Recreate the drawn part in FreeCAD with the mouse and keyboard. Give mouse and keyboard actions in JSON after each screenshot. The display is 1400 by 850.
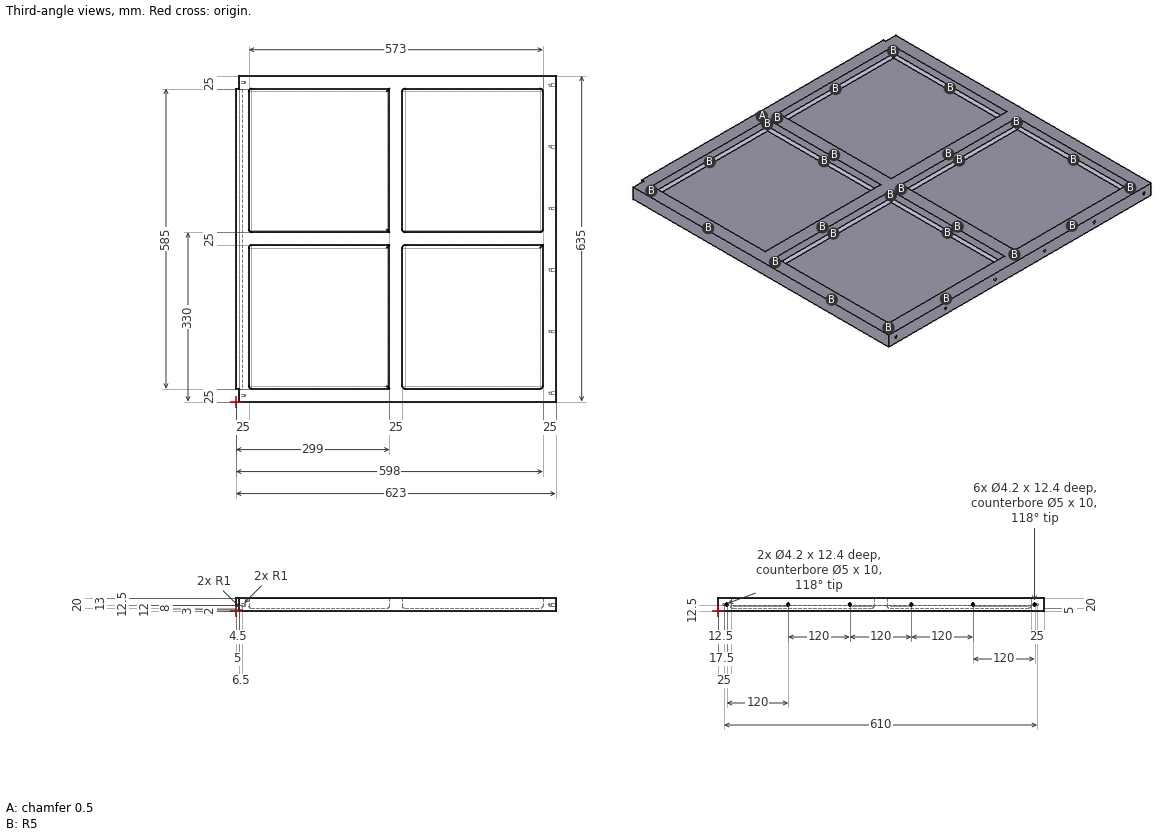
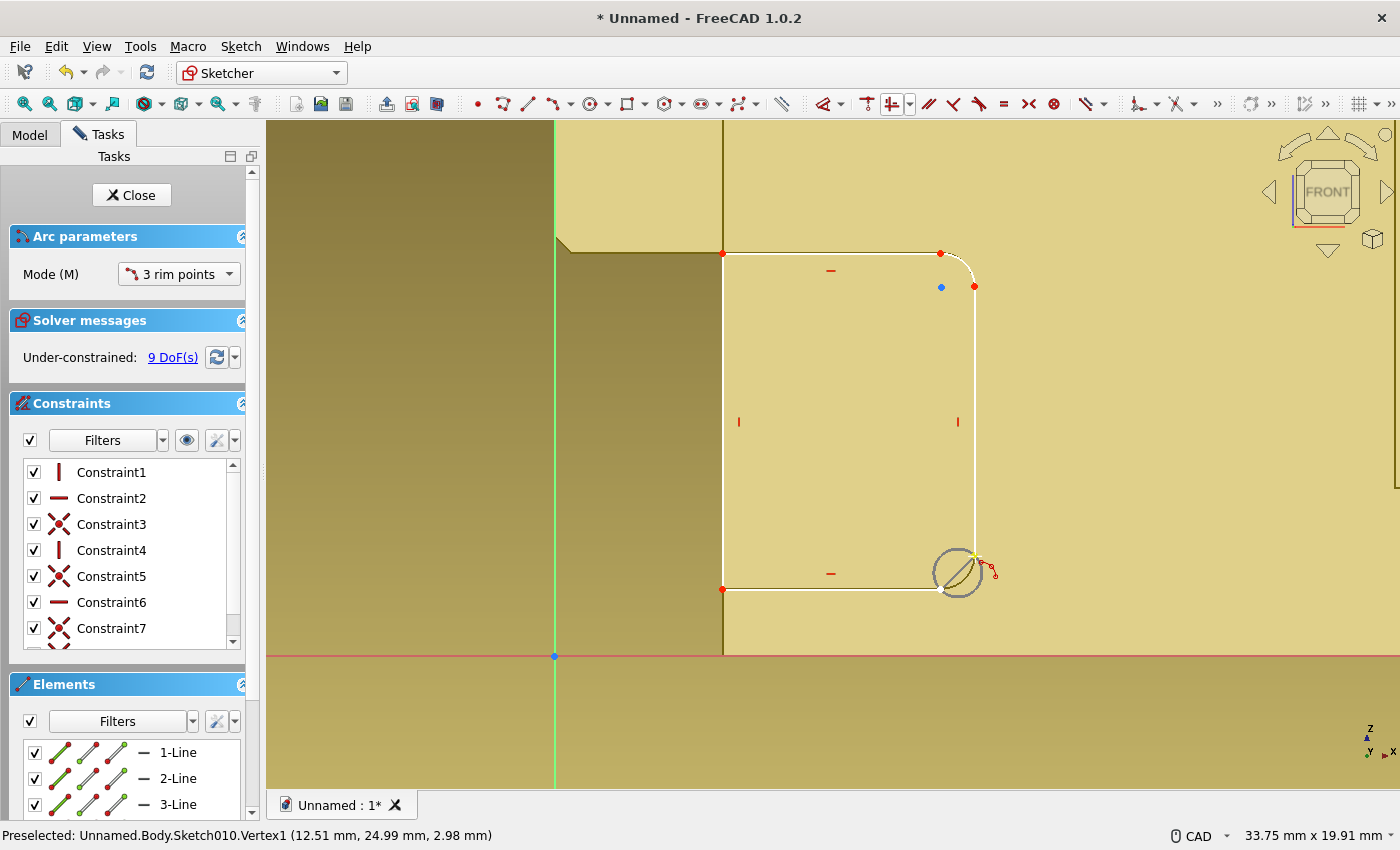
{"action": "scroll", "coordinate": [965, 579], "scroll_direction": "up", "scroll_amount": 3}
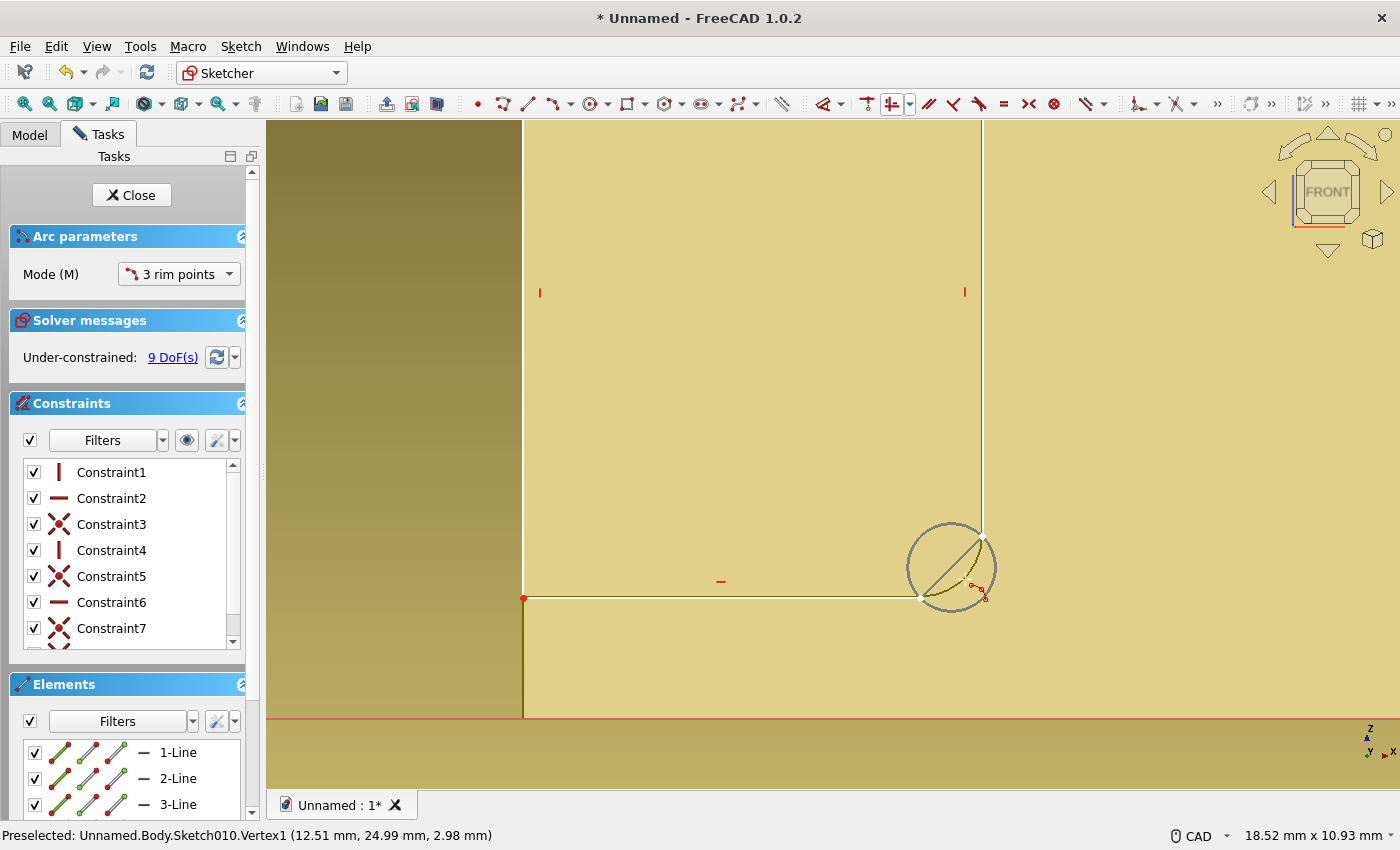
{"action": "left_click", "coordinate": [964, 579]}
{"action": "key", "text": "Escape"}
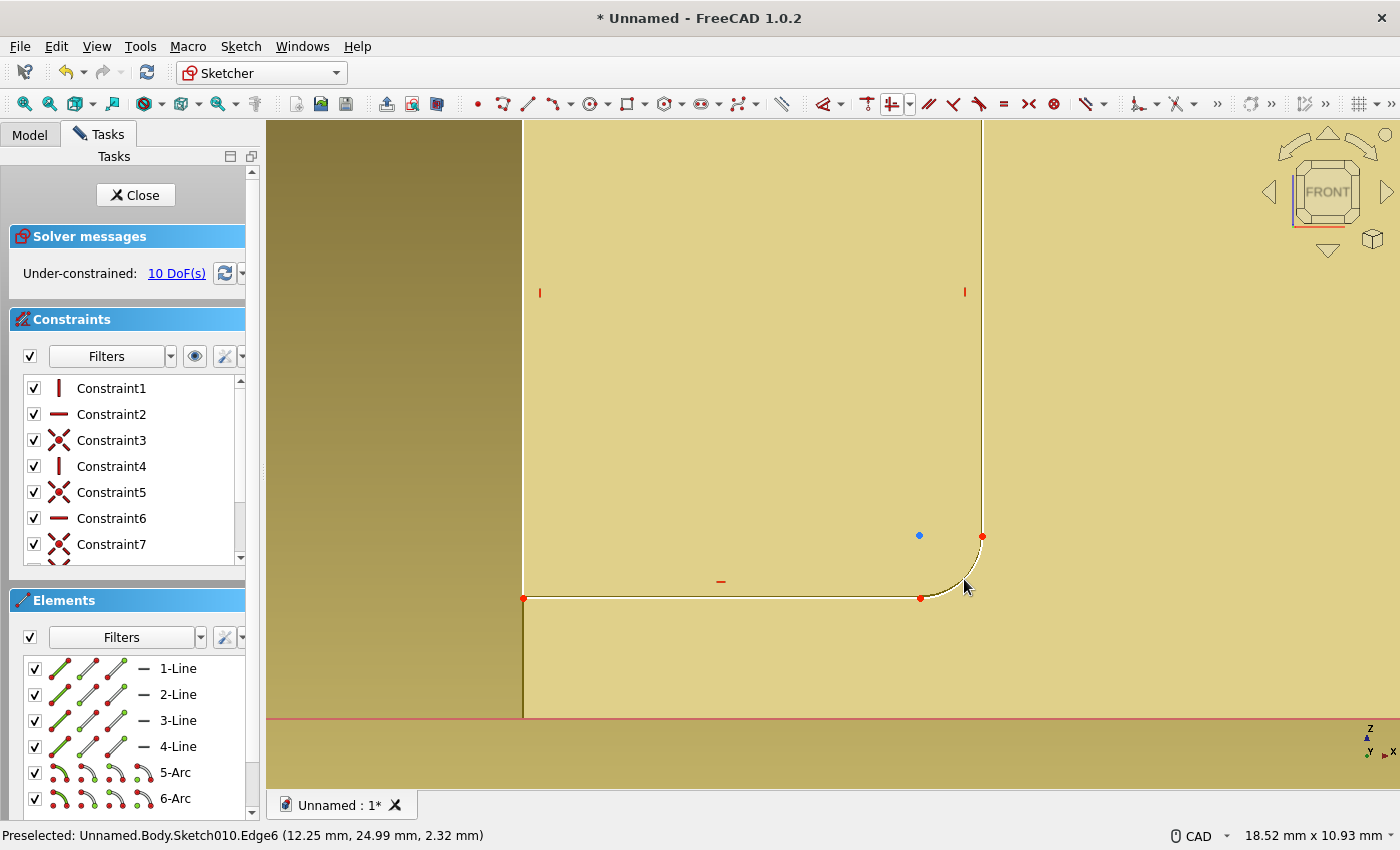
{"action": "left_click", "coordinate": [983, 389]}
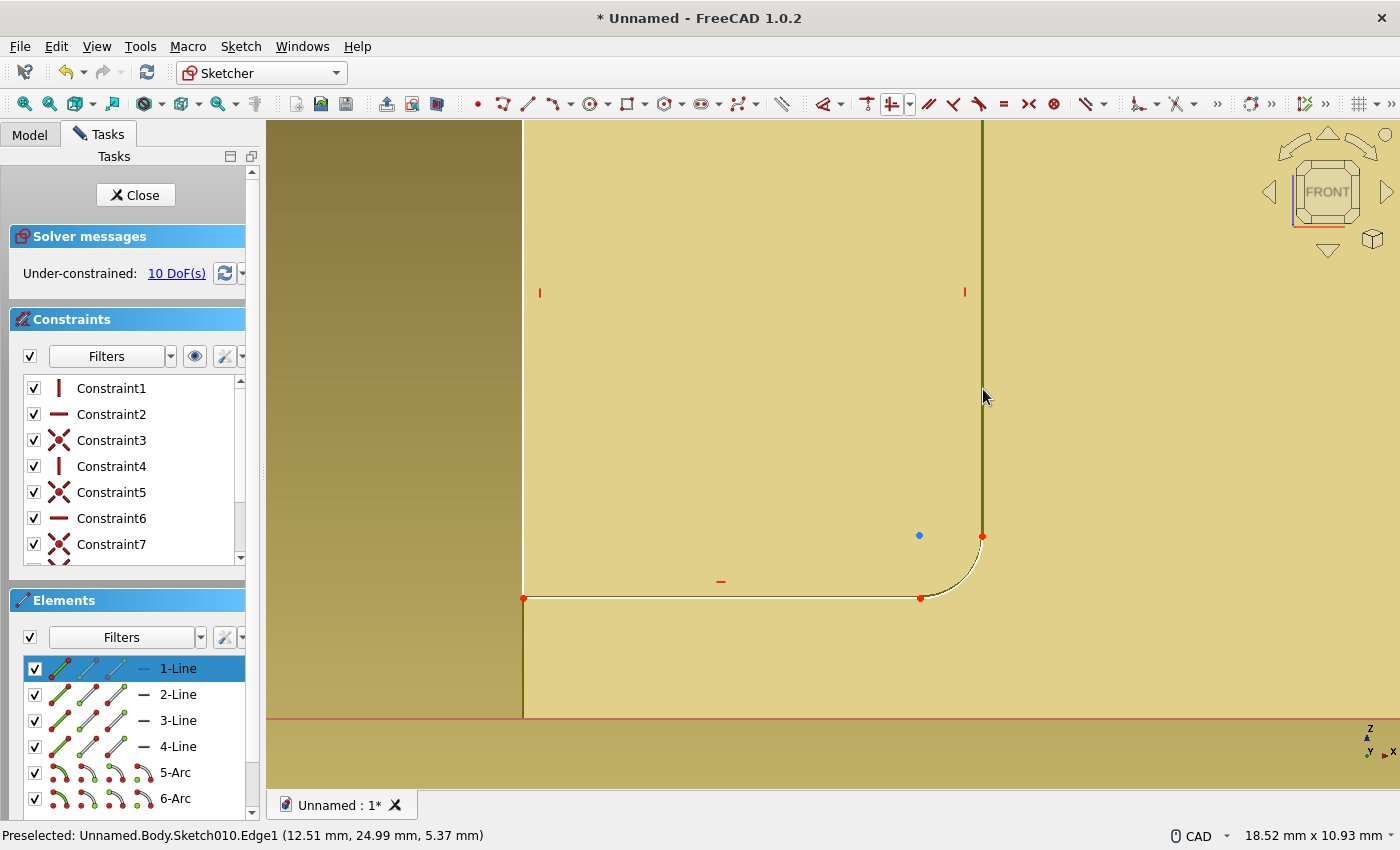
{"action": "scroll", "coordinate": [965, 580], "scroll_direction": "down", "scroll_amount": 3}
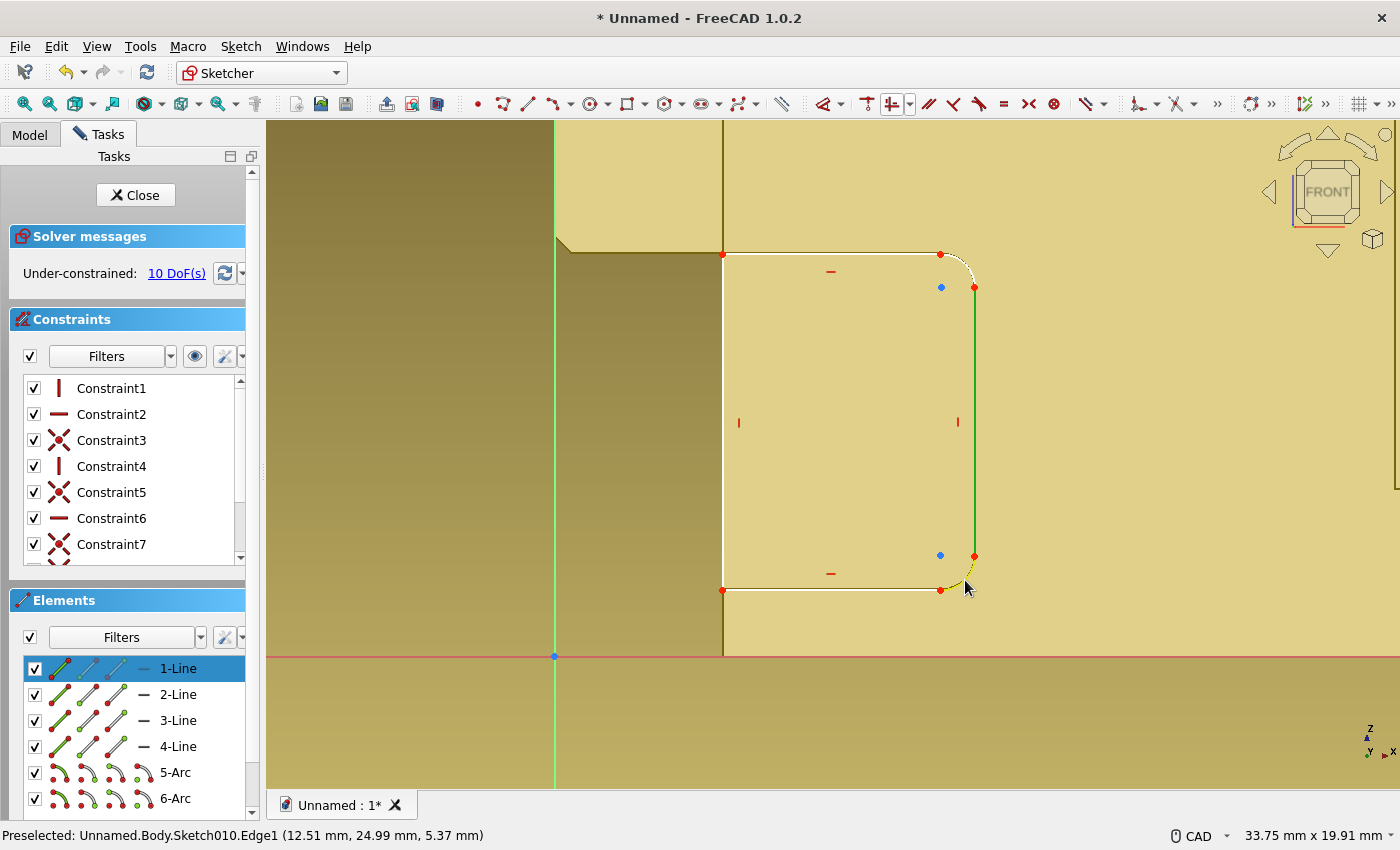
{"action": "left_click", "coordinate": [971, 272]}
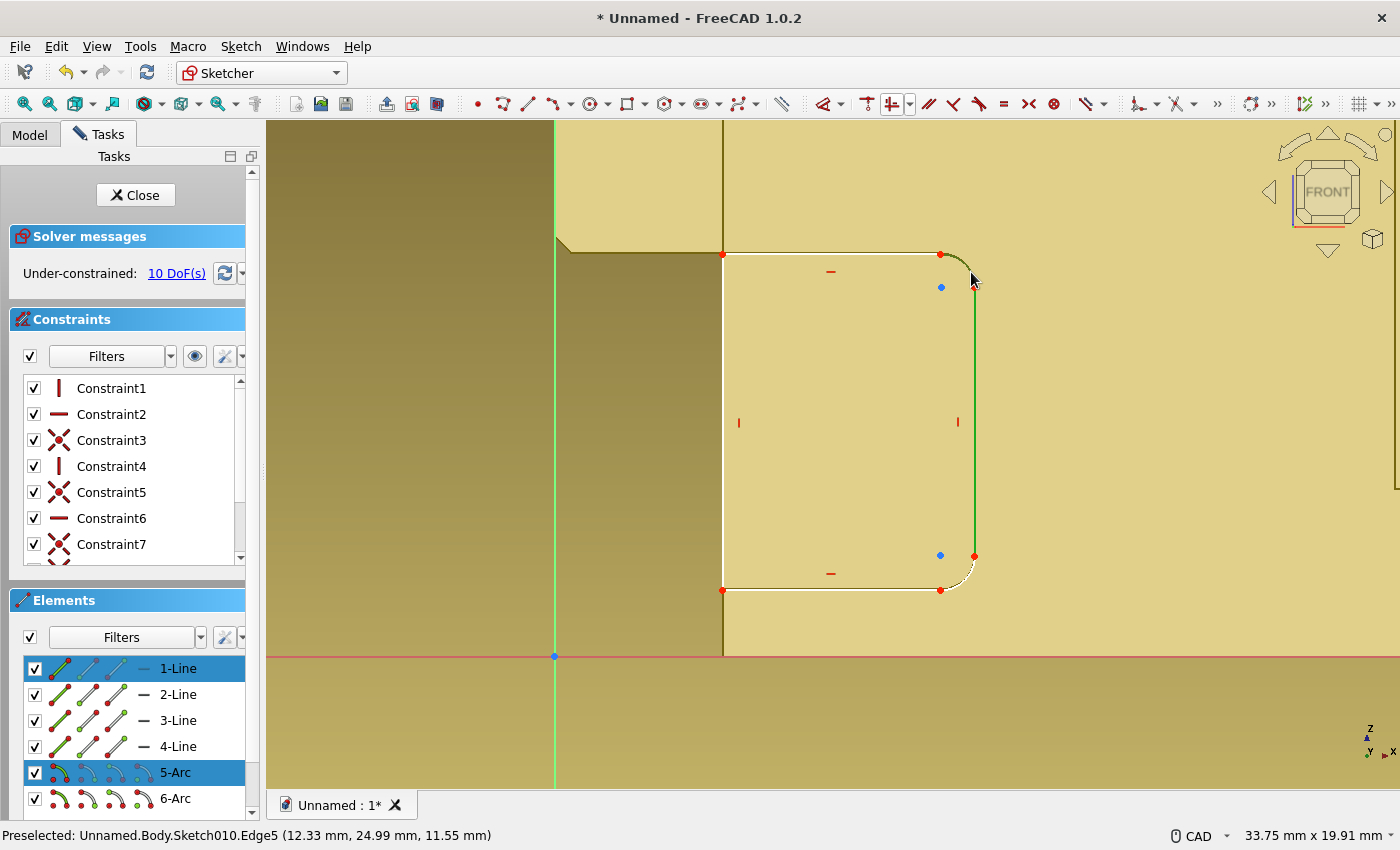
{"action": "left_click", "coordinate": [979, 104]}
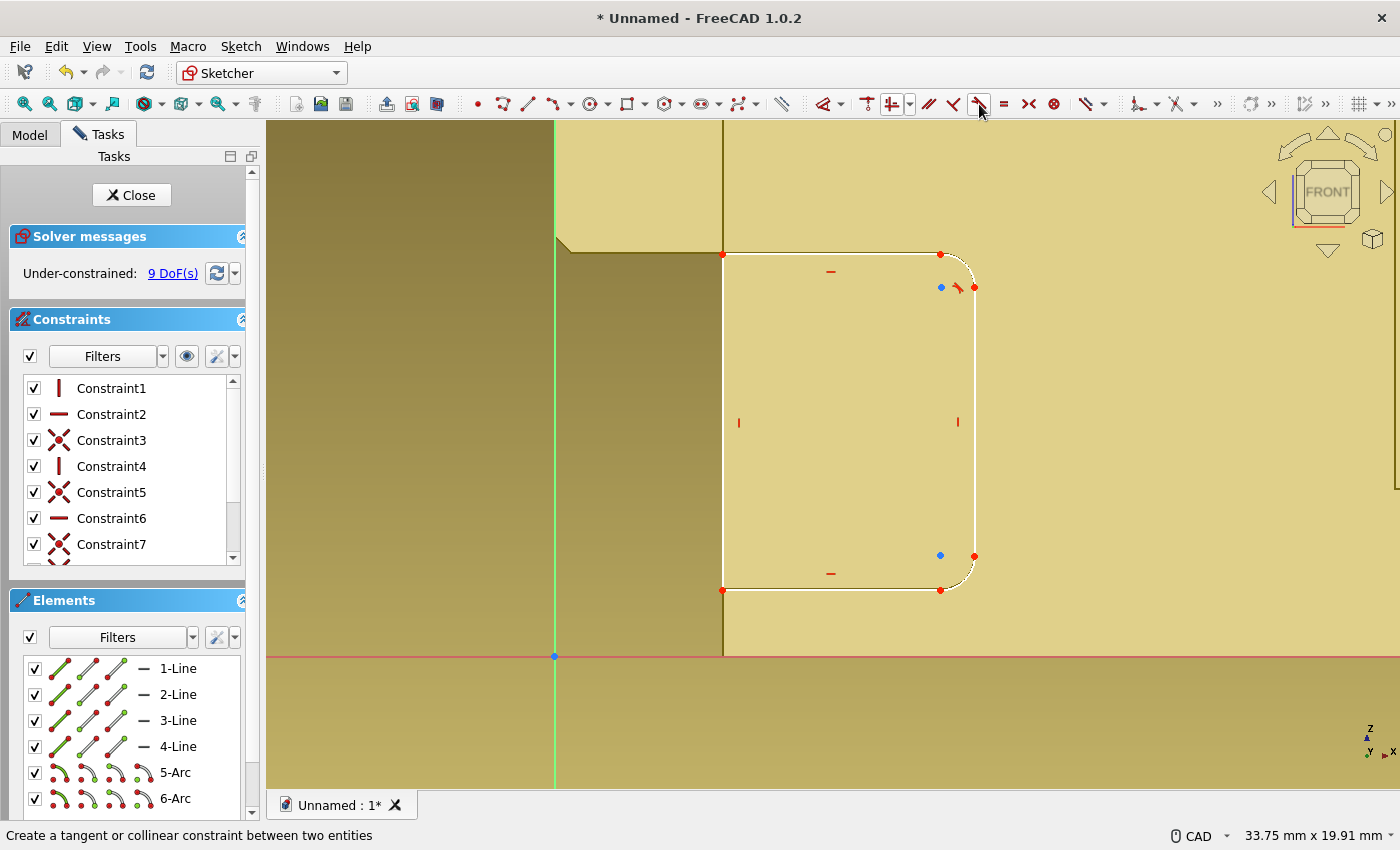
{"action": "left_click", "coordinate": [975, 476]}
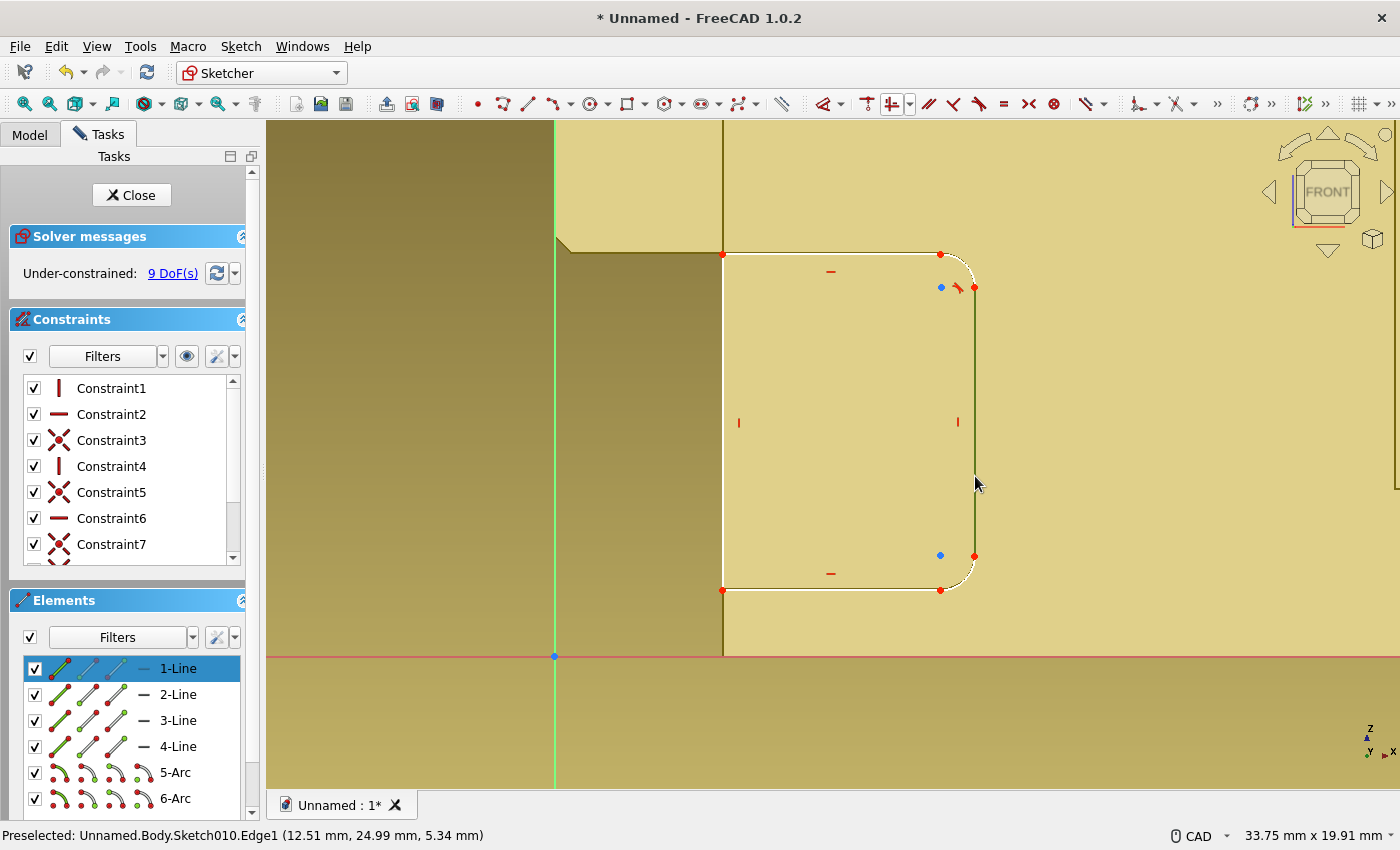
{"action": "left_click", "coordinate": [956, 587]}